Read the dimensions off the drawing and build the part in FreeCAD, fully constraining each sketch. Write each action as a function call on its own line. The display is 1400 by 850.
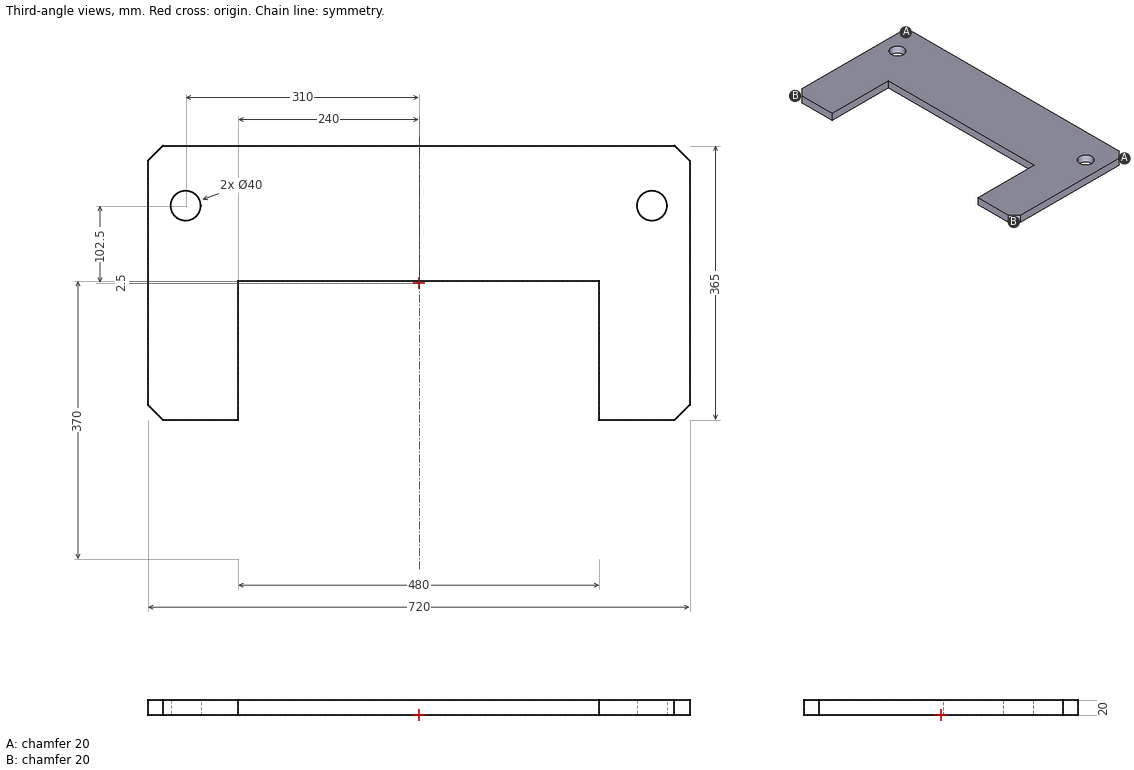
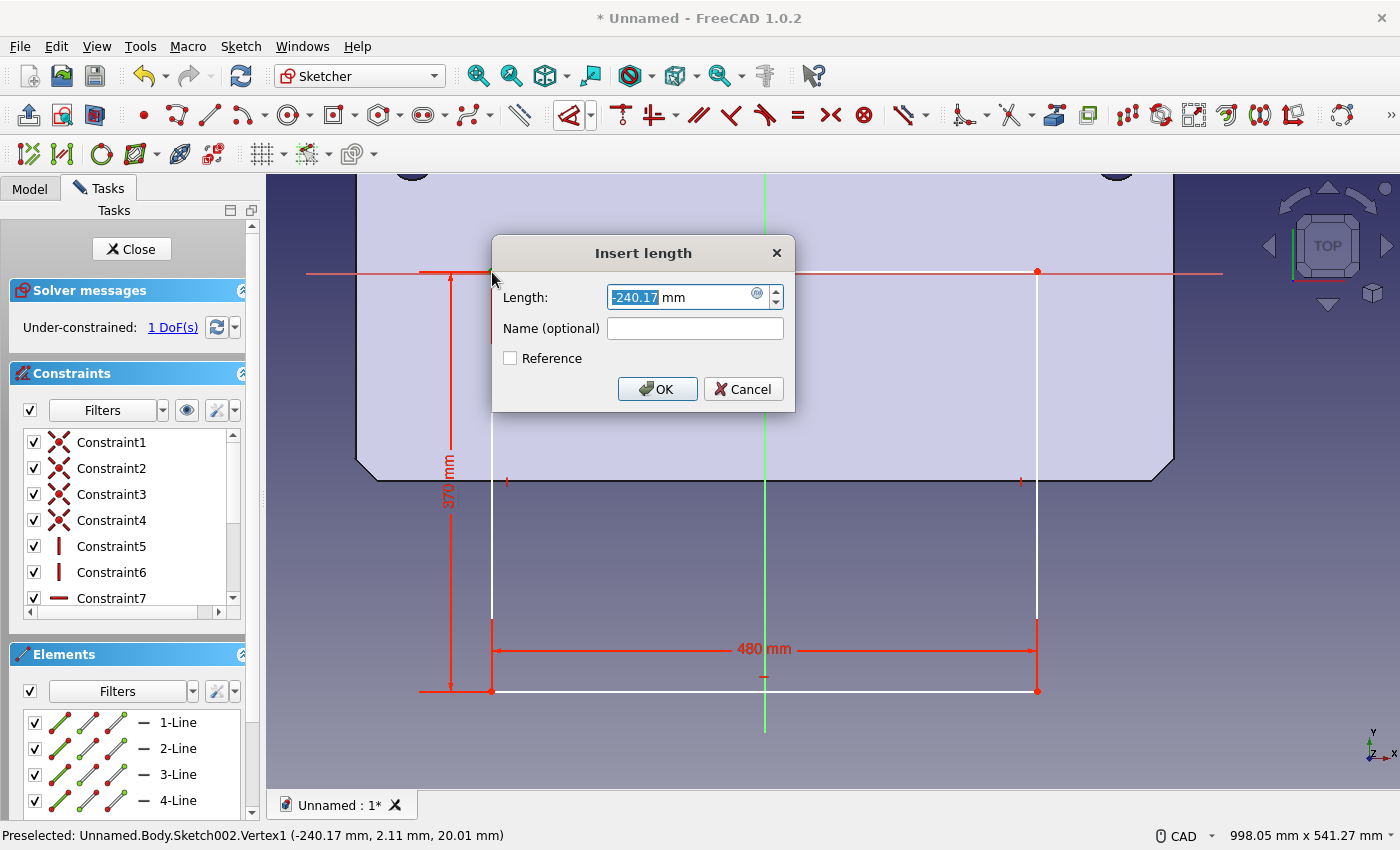
text(-240)
key(Return)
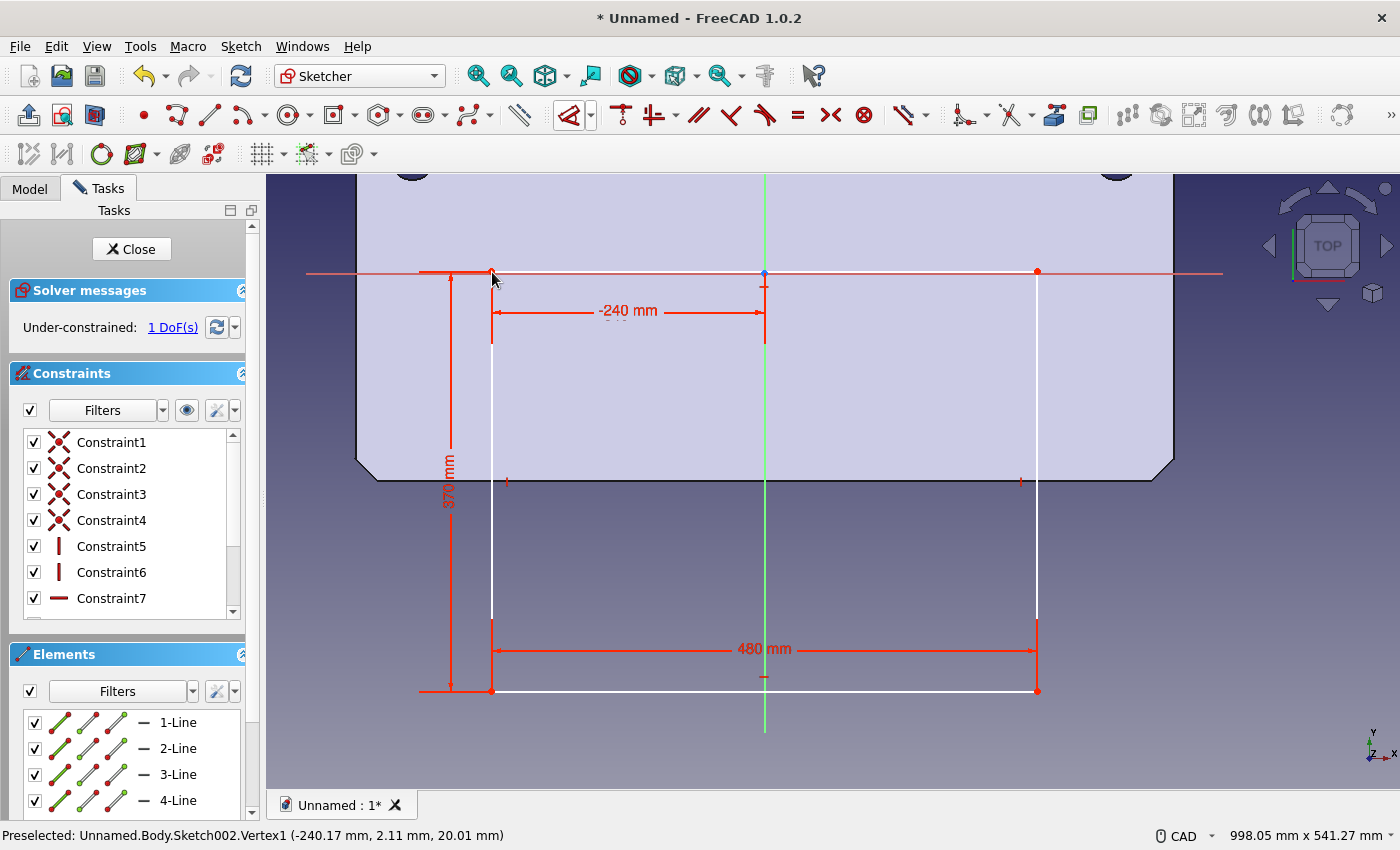
scroll(492, 272, up, 14)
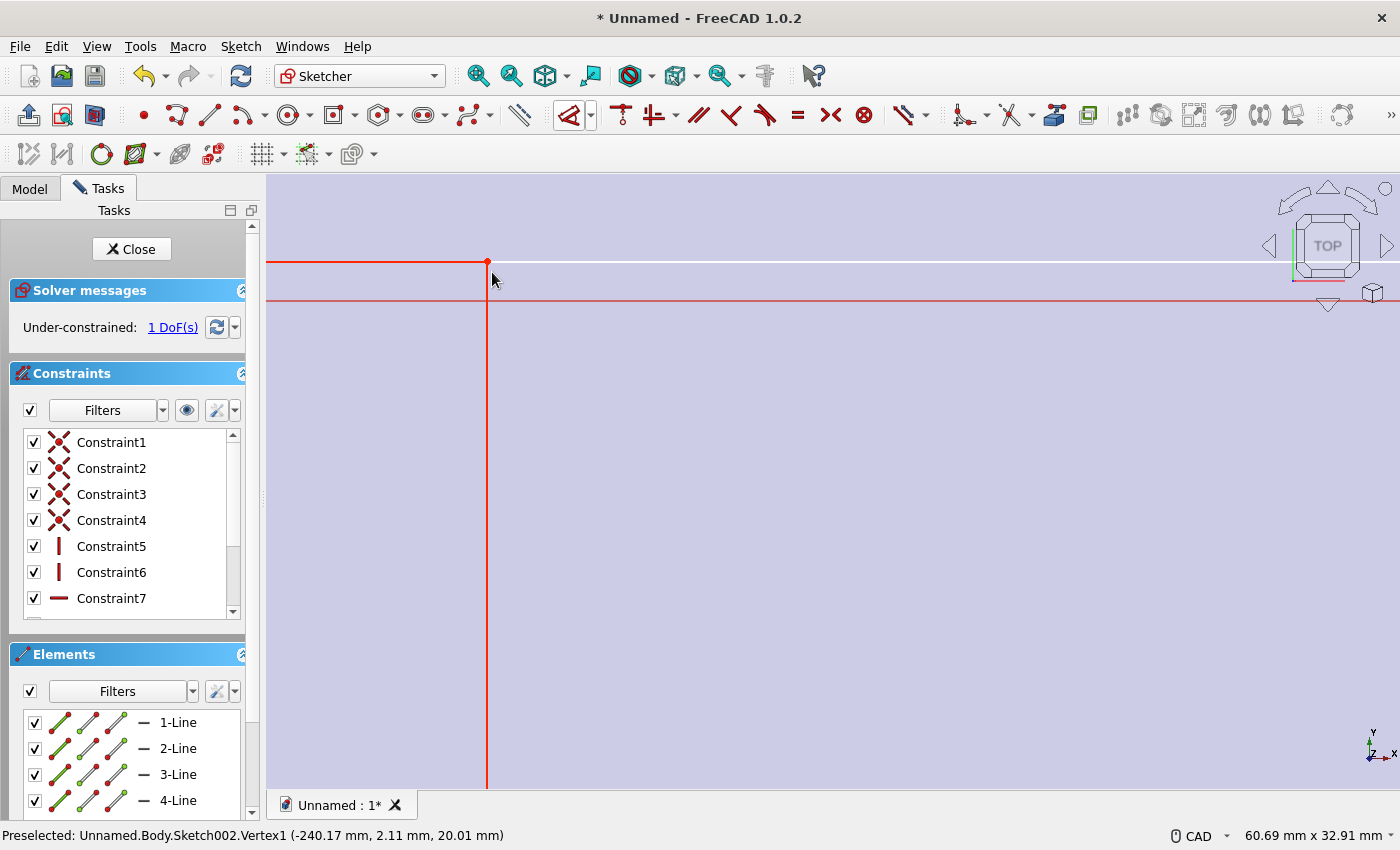
click(487, 262)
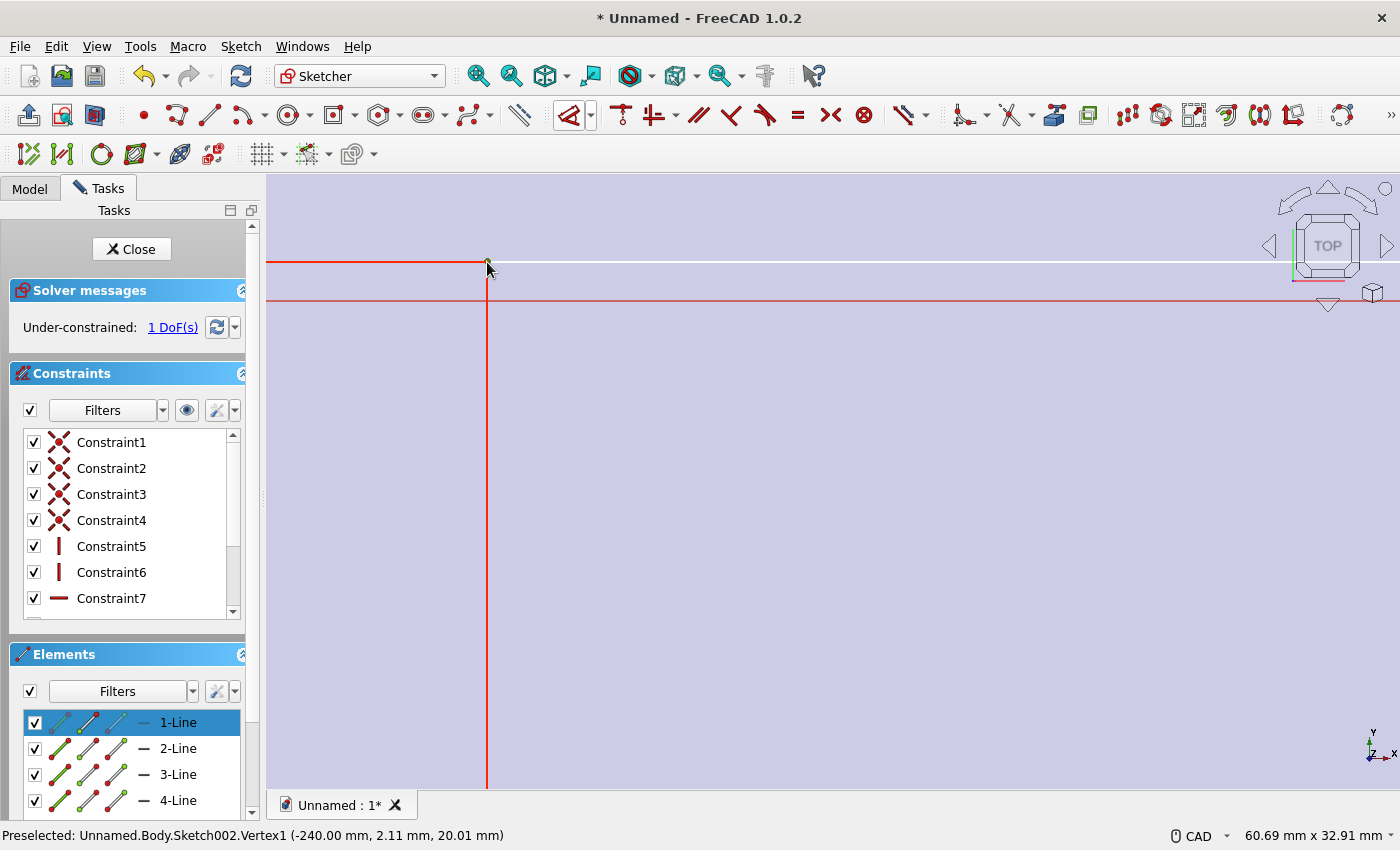
key(i)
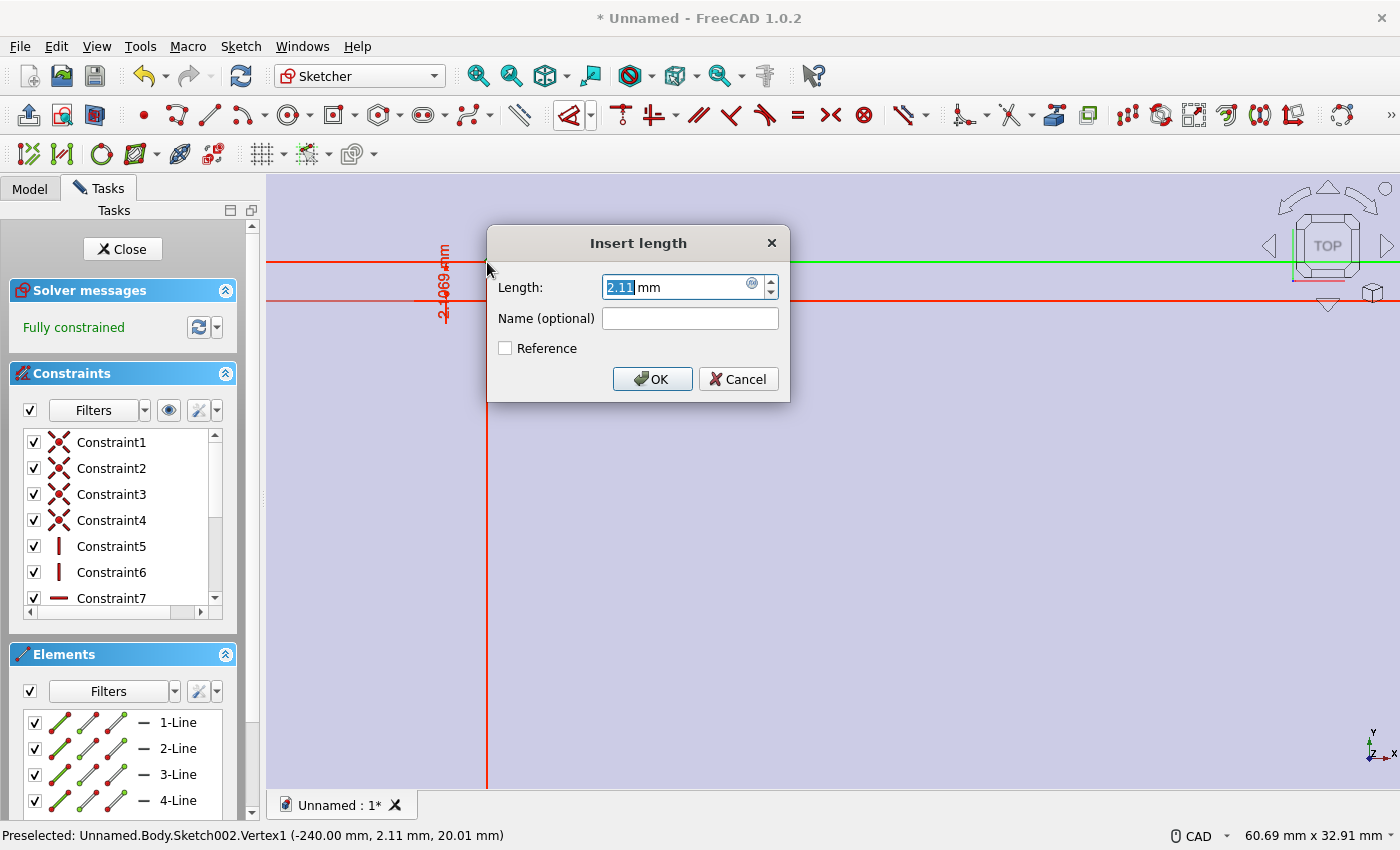
text(2.5)
key(Return)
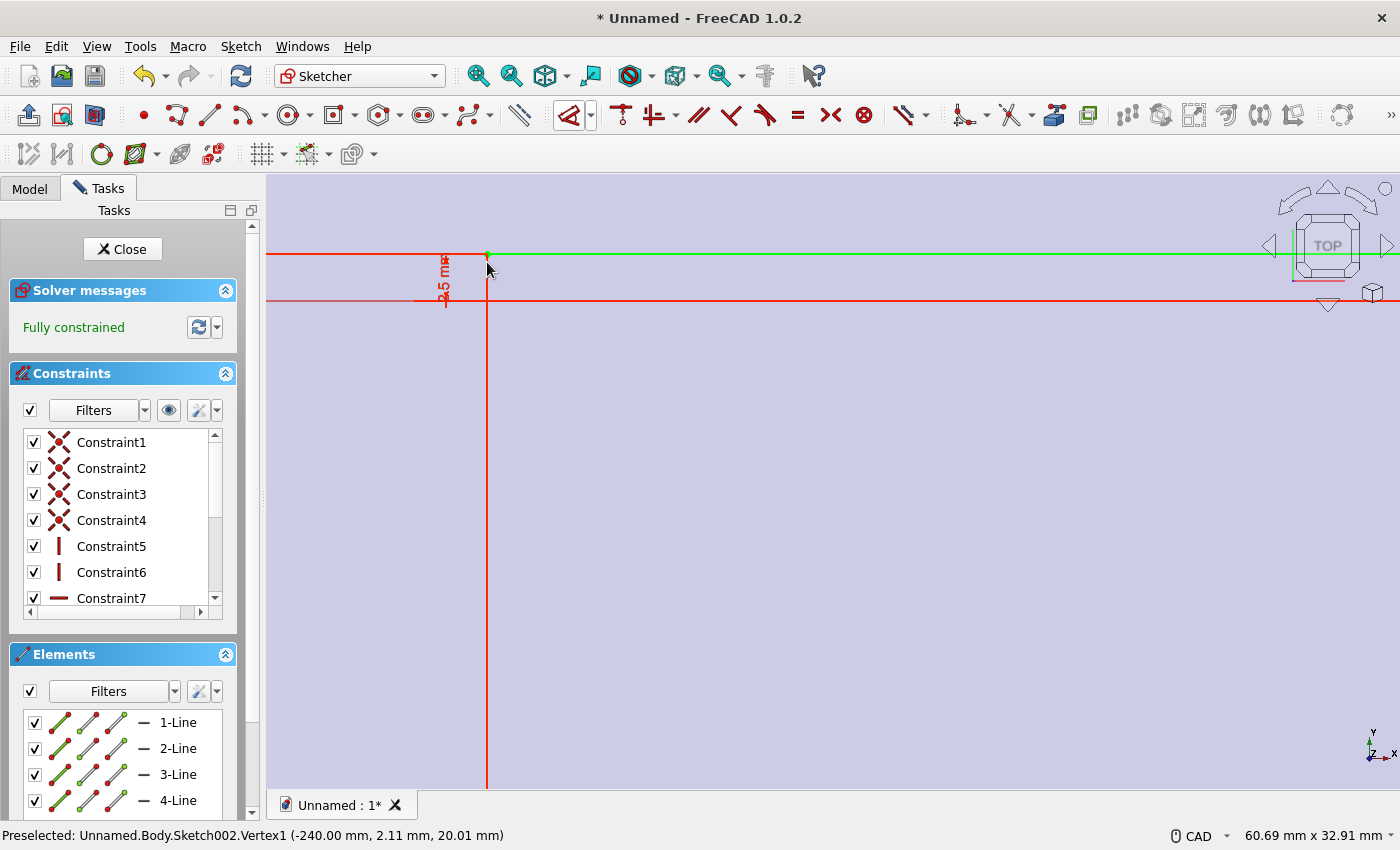
click(123, 249)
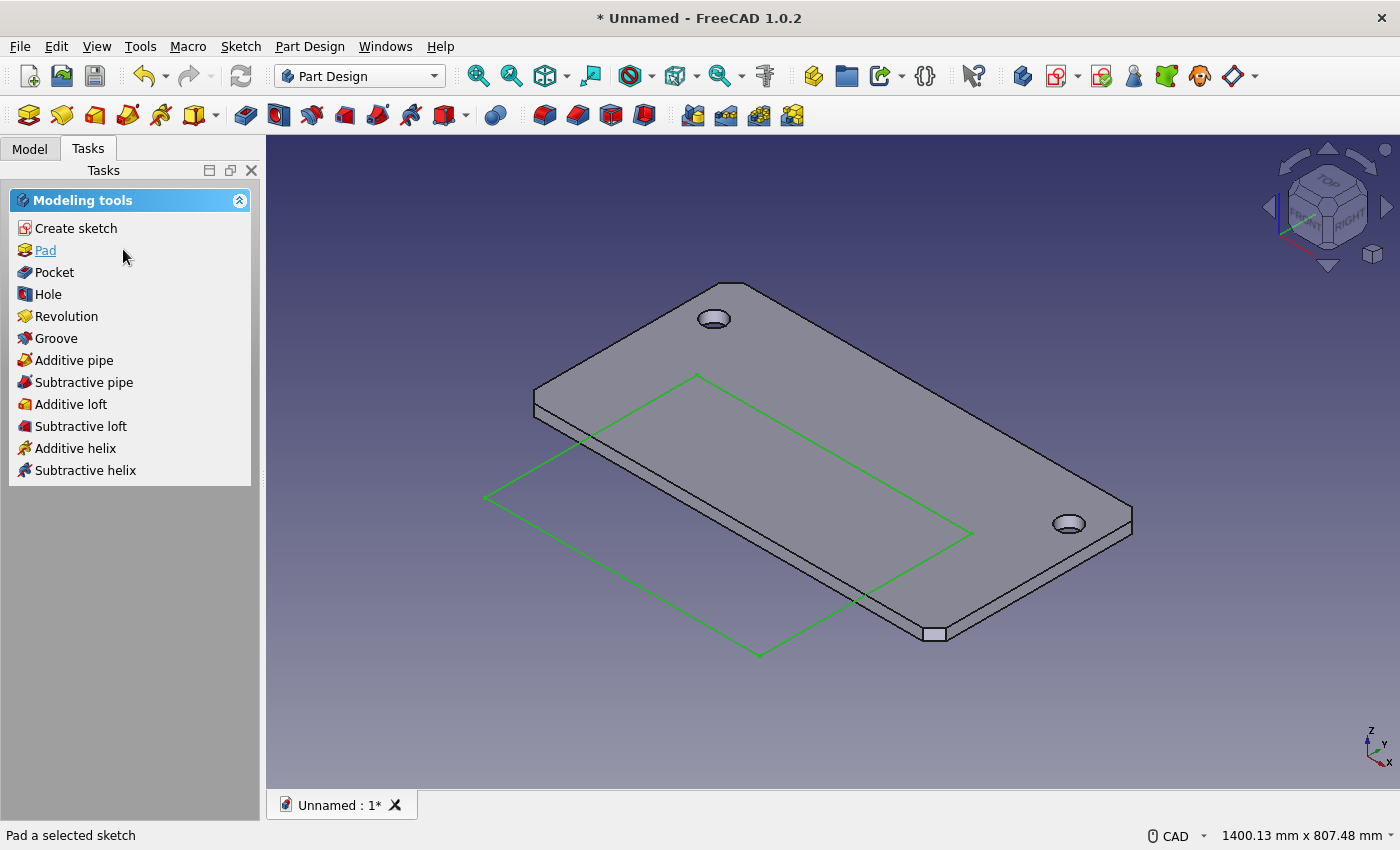
click(246, 116)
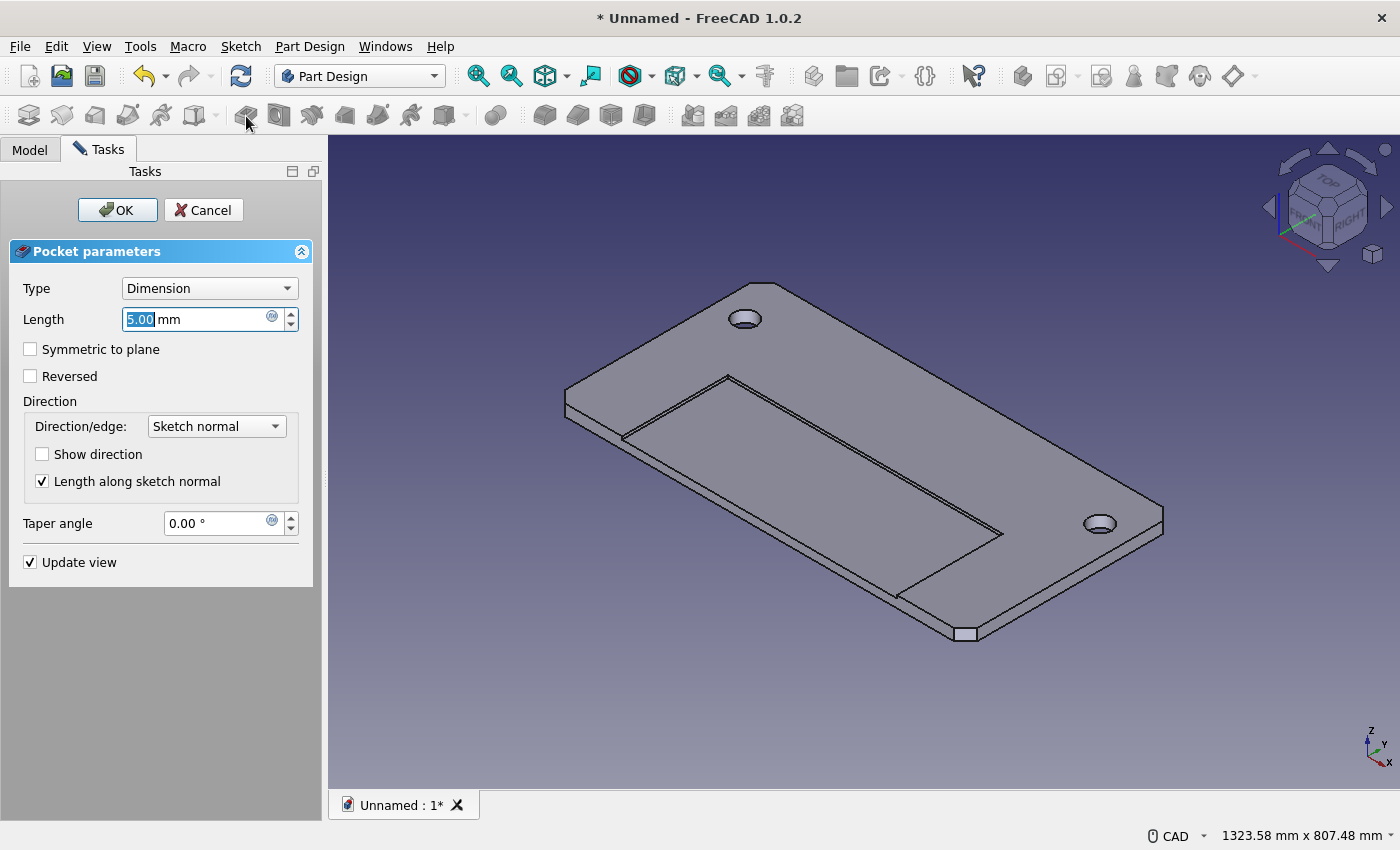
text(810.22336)
key(Tab)